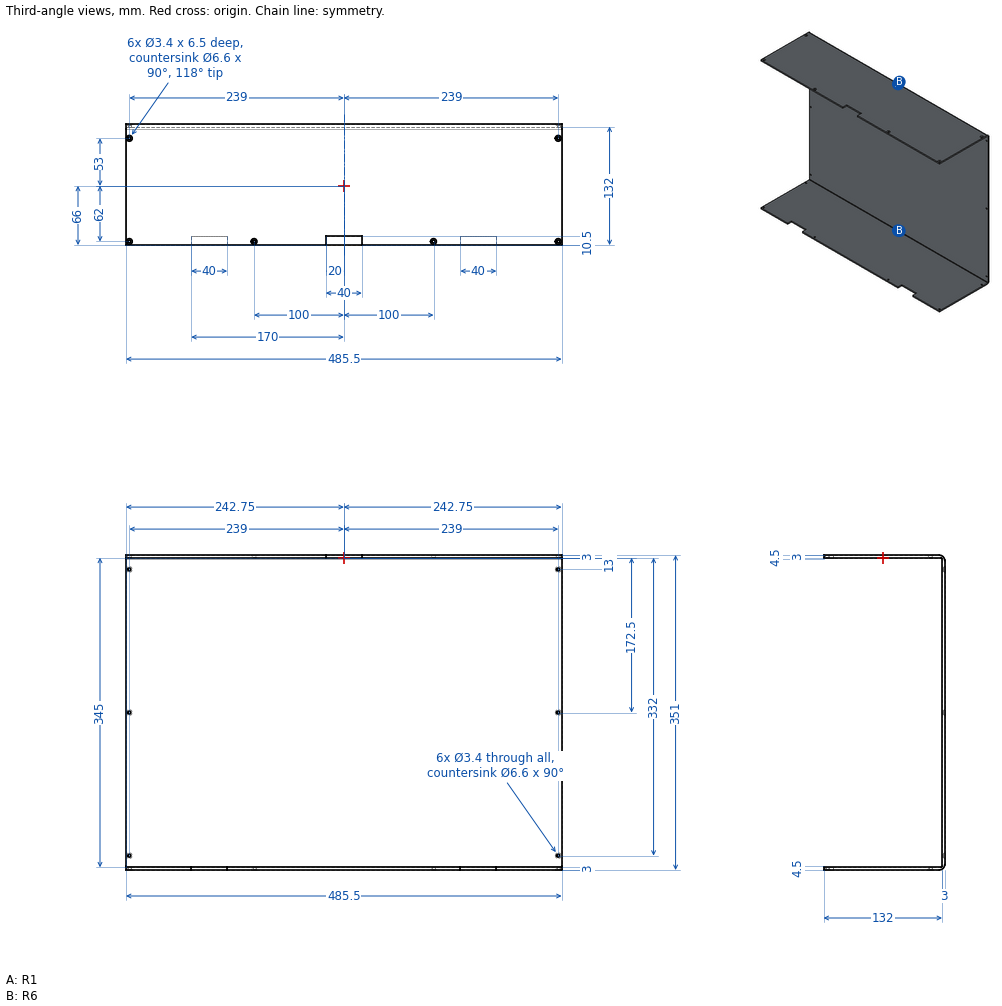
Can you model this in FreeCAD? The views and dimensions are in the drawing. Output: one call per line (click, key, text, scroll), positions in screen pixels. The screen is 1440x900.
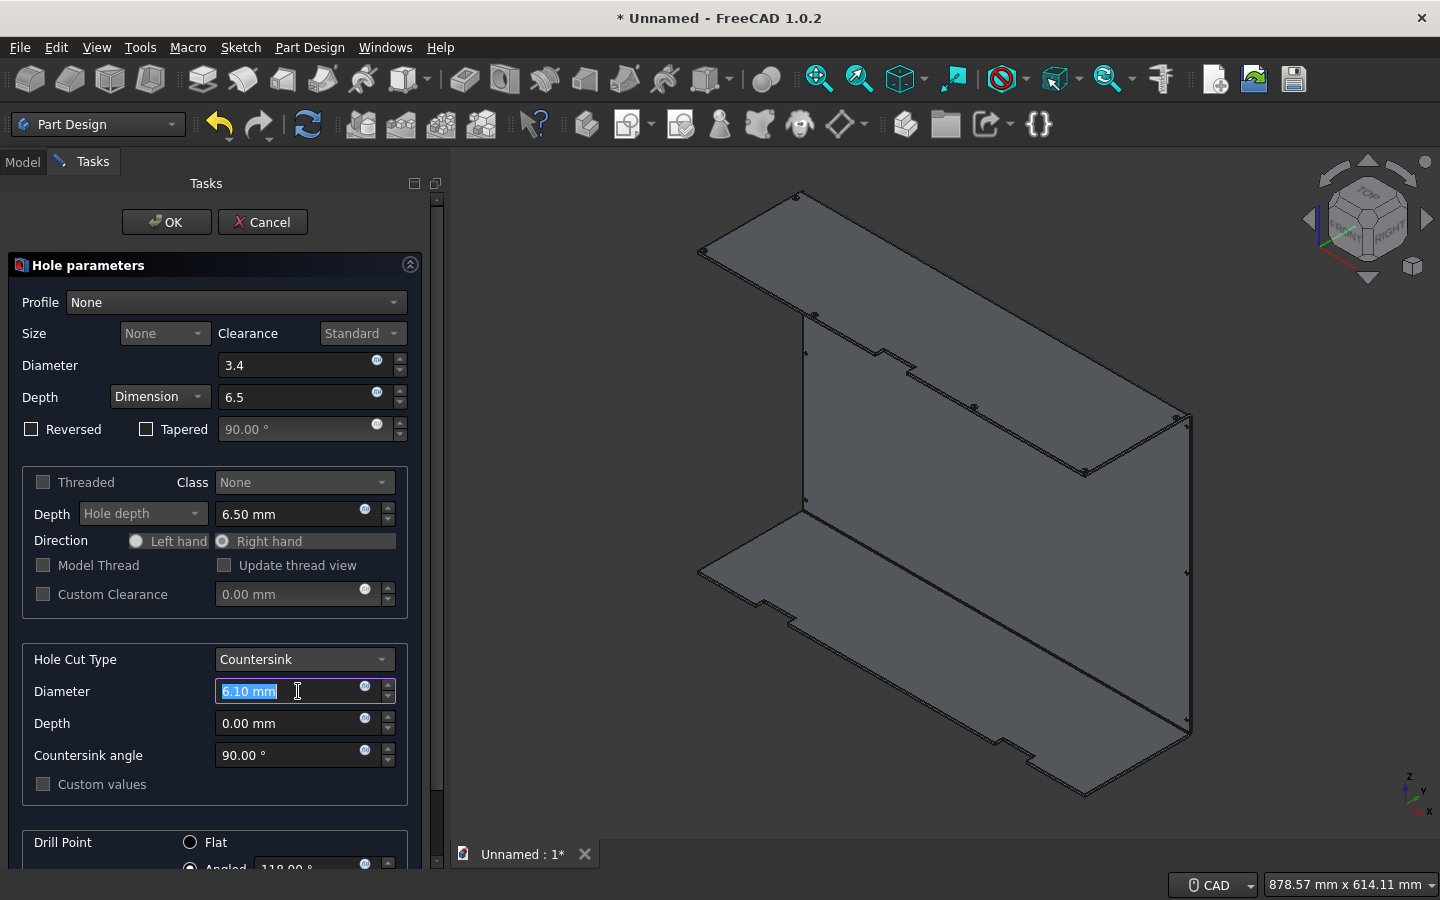
text(6.6)
key(Tab)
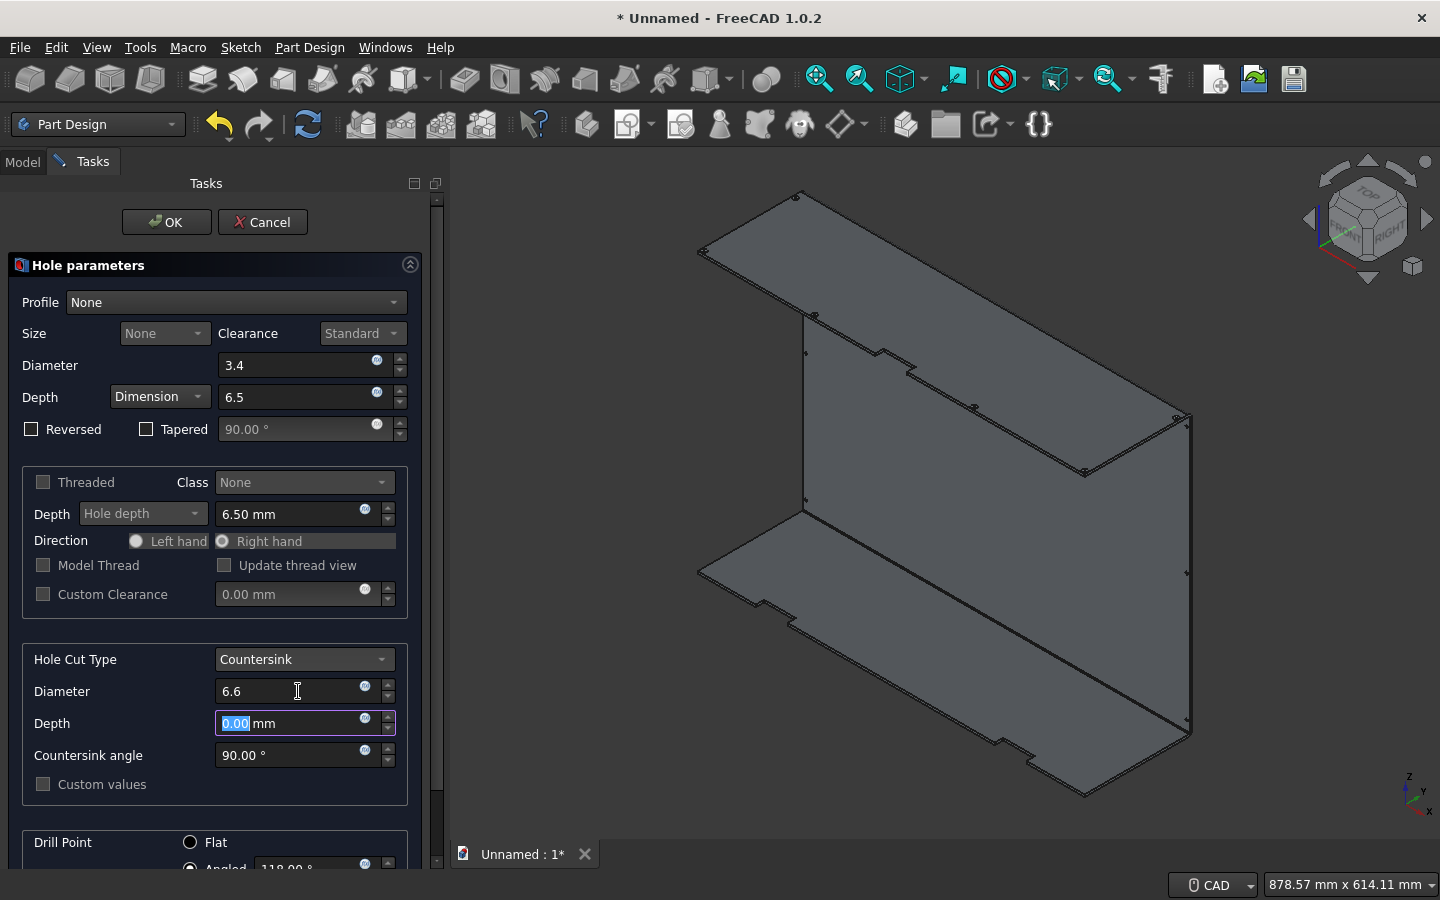
click(167, 222)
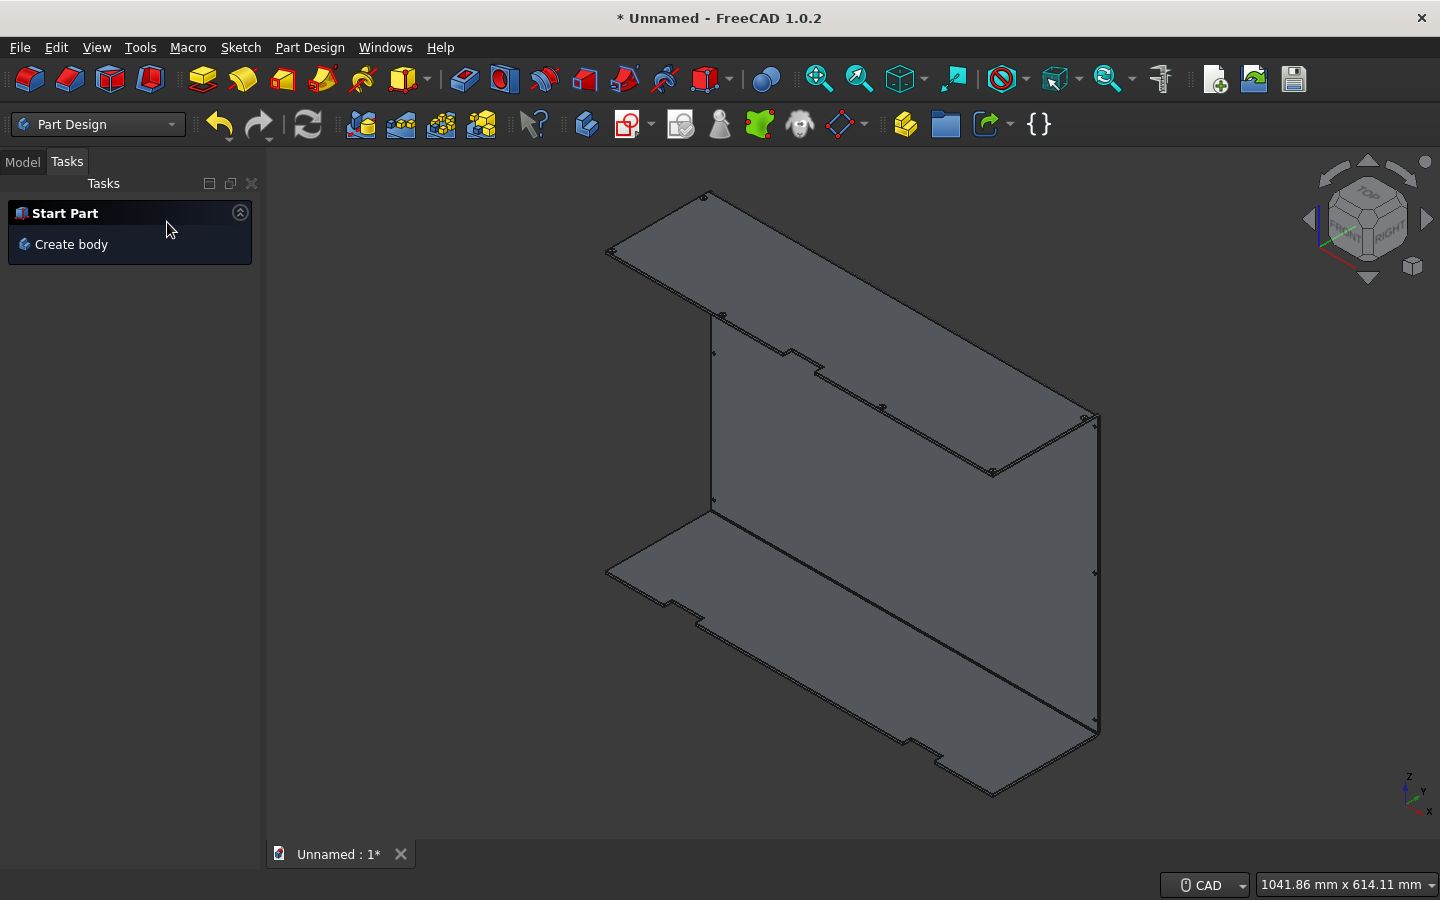
key(5)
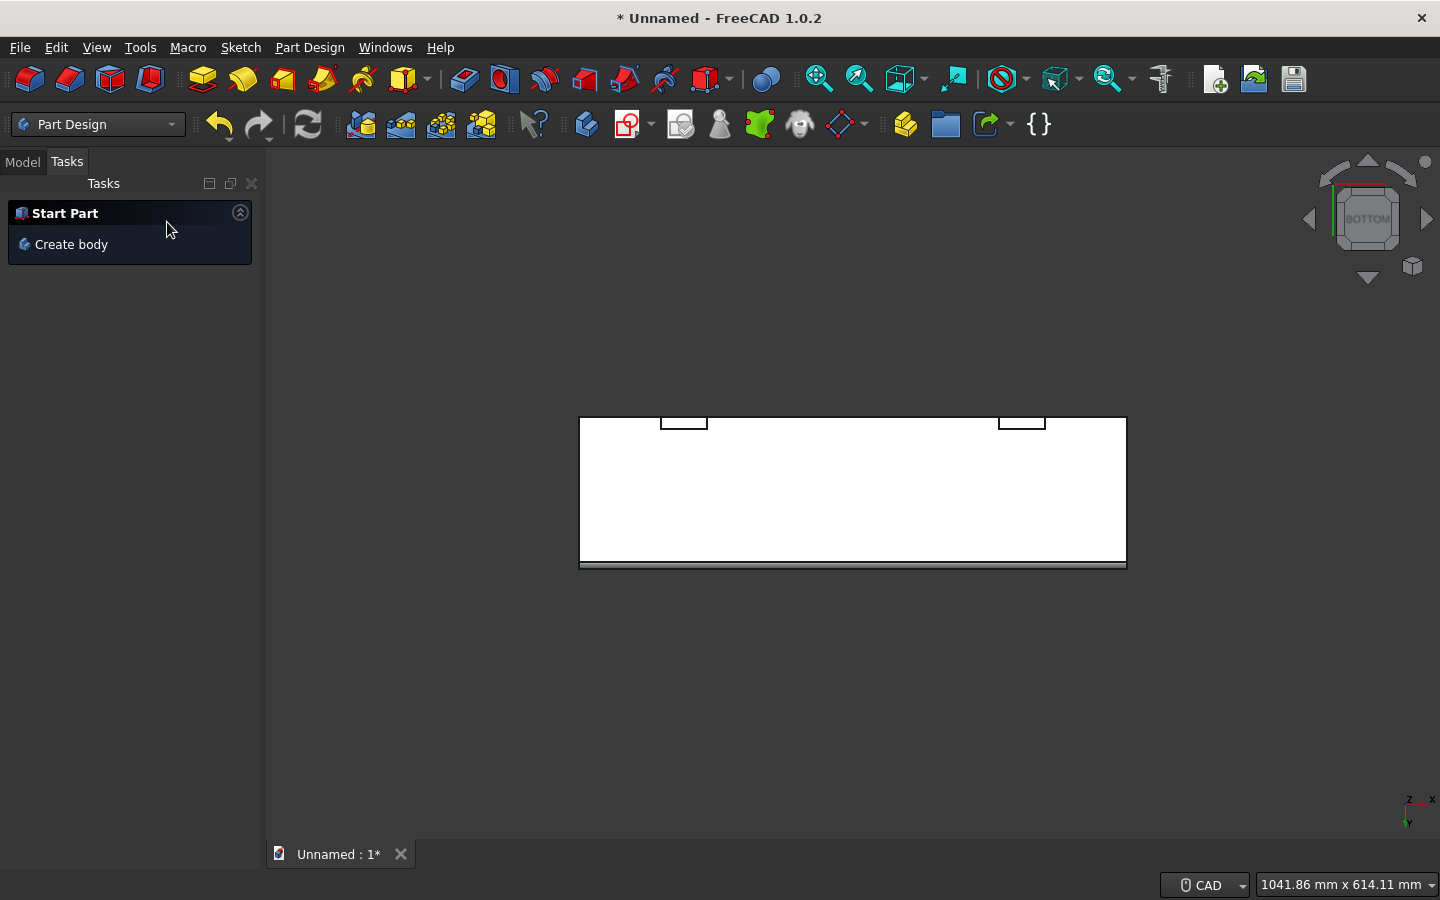
click(931, 489)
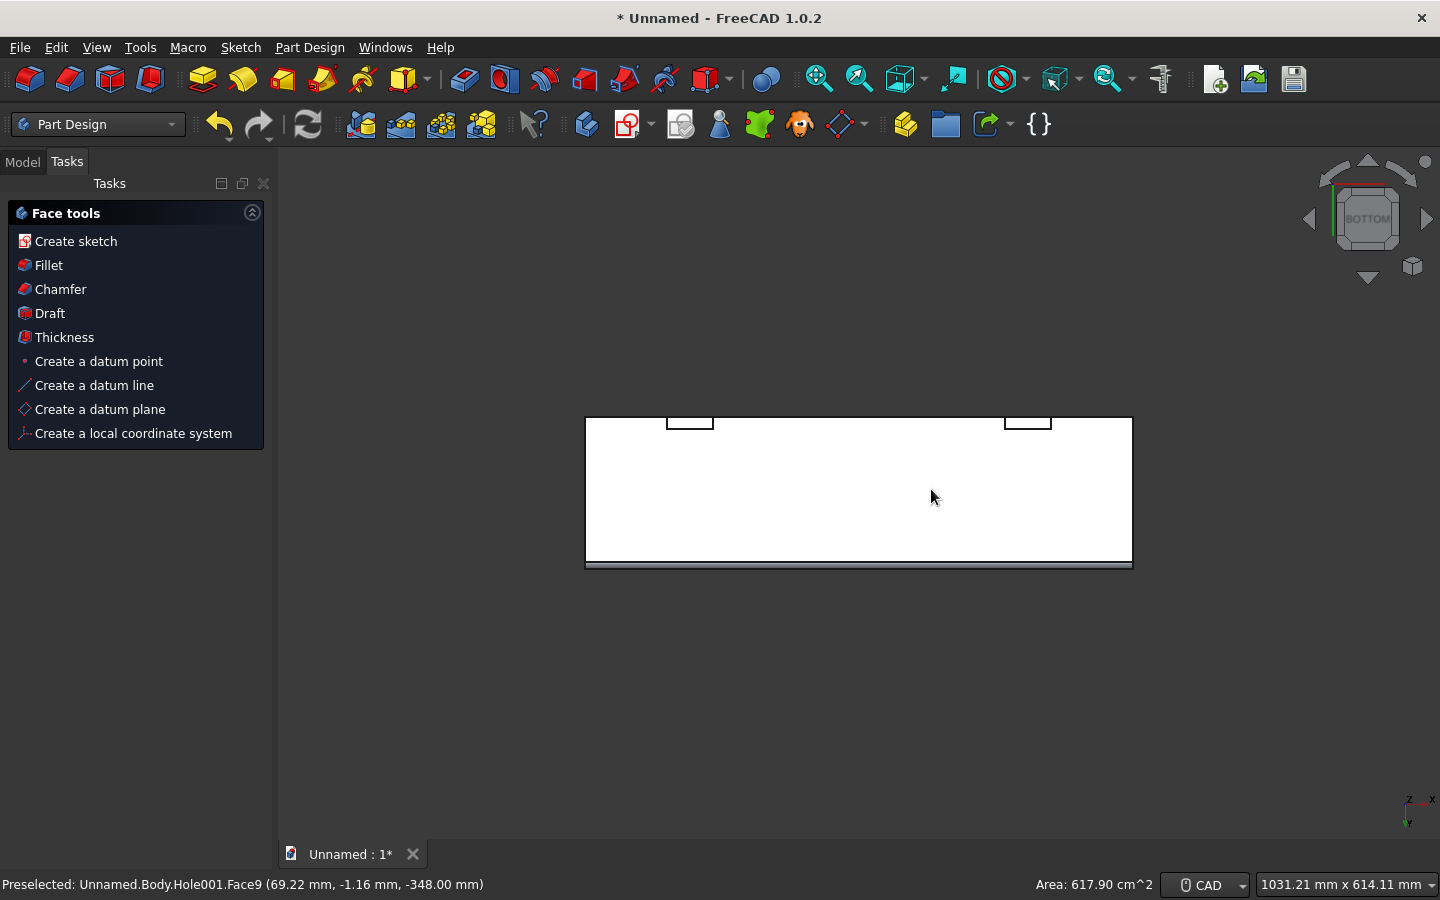
click(628, 124)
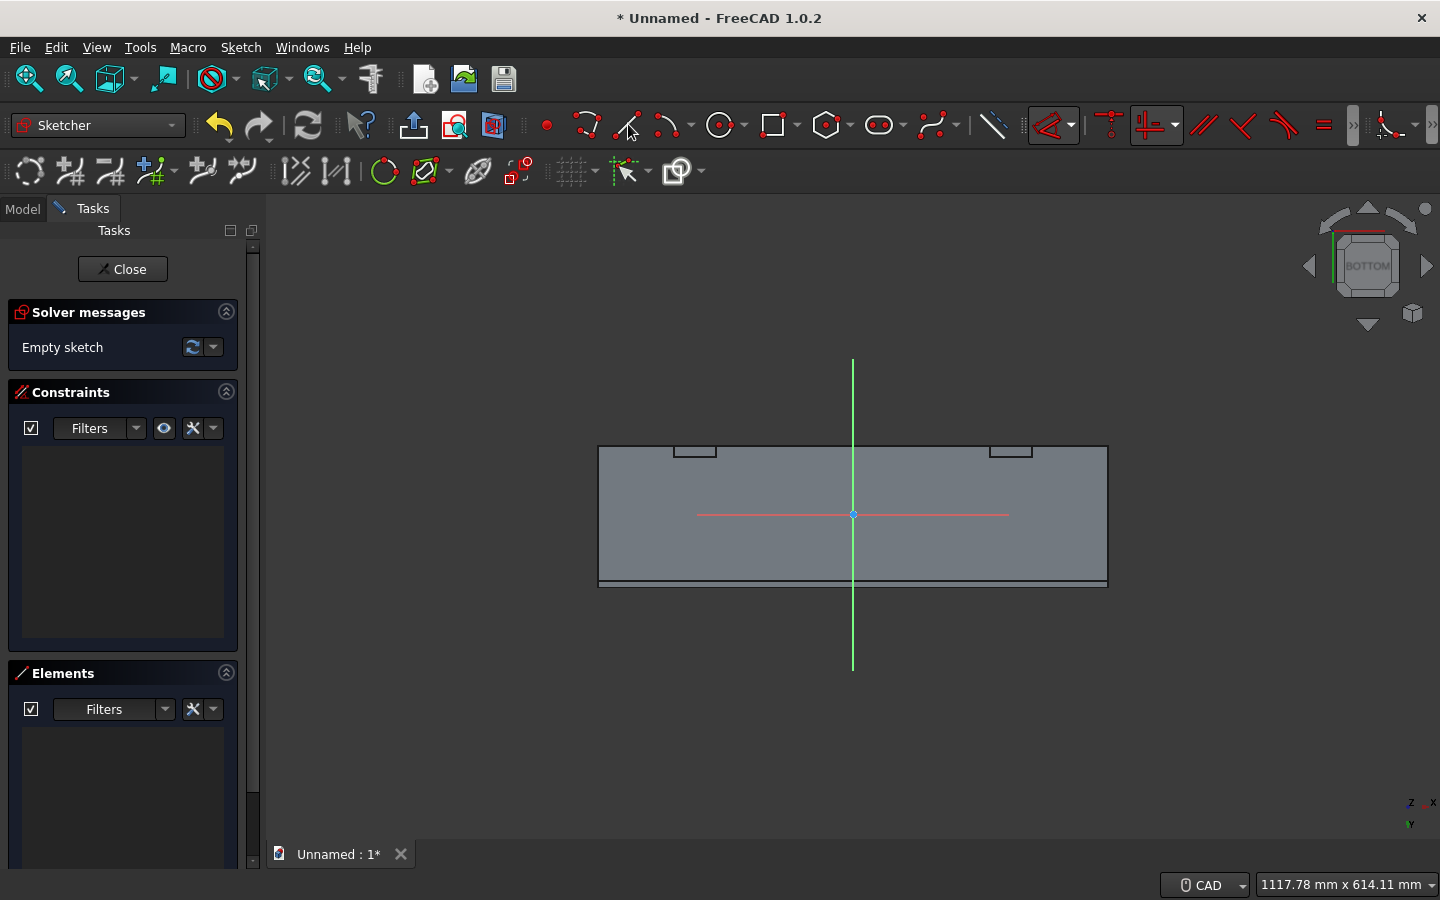
scroll(992, 497, up, 2)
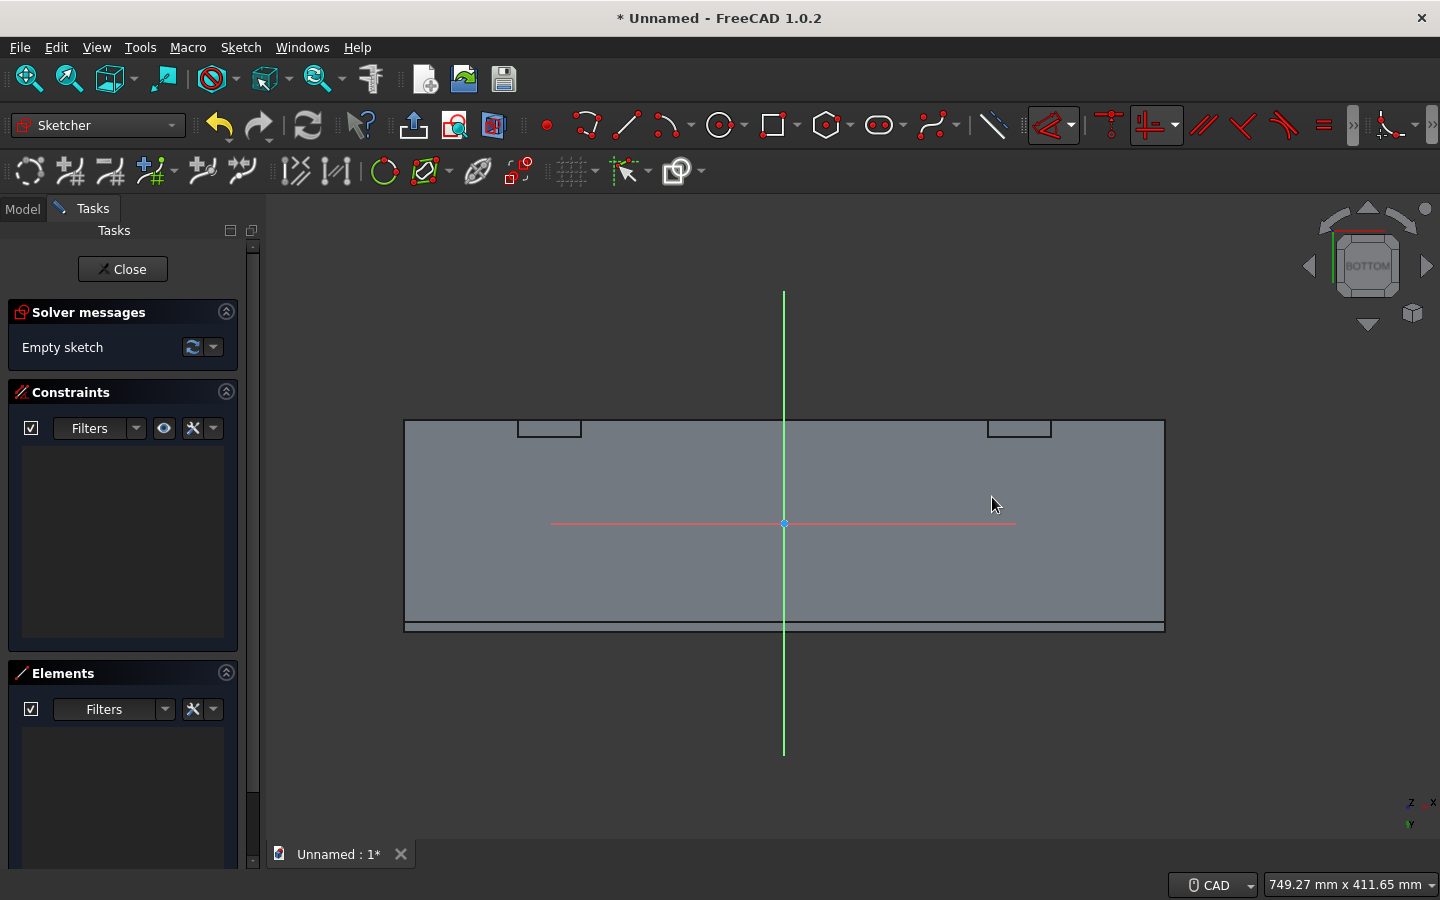
click(720, 126)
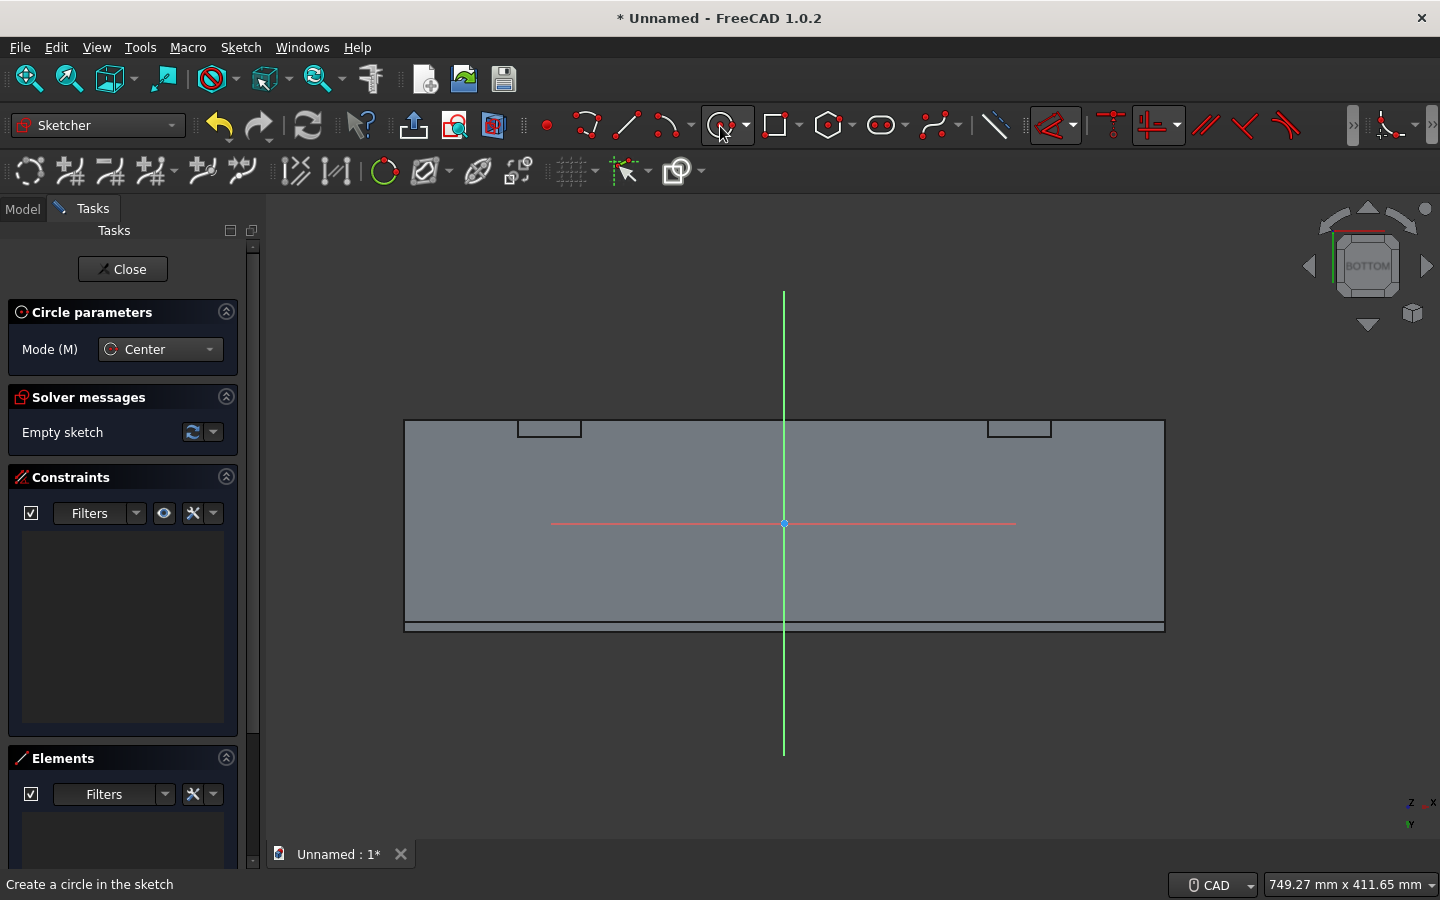
scroll(410, 607, up, 11)